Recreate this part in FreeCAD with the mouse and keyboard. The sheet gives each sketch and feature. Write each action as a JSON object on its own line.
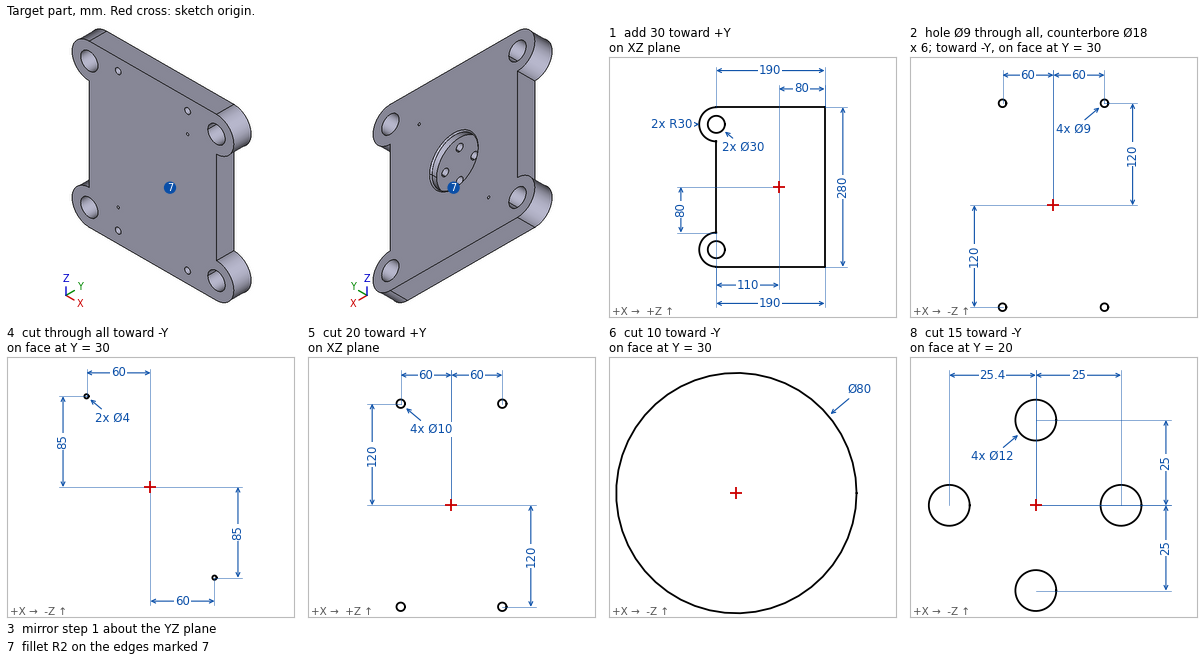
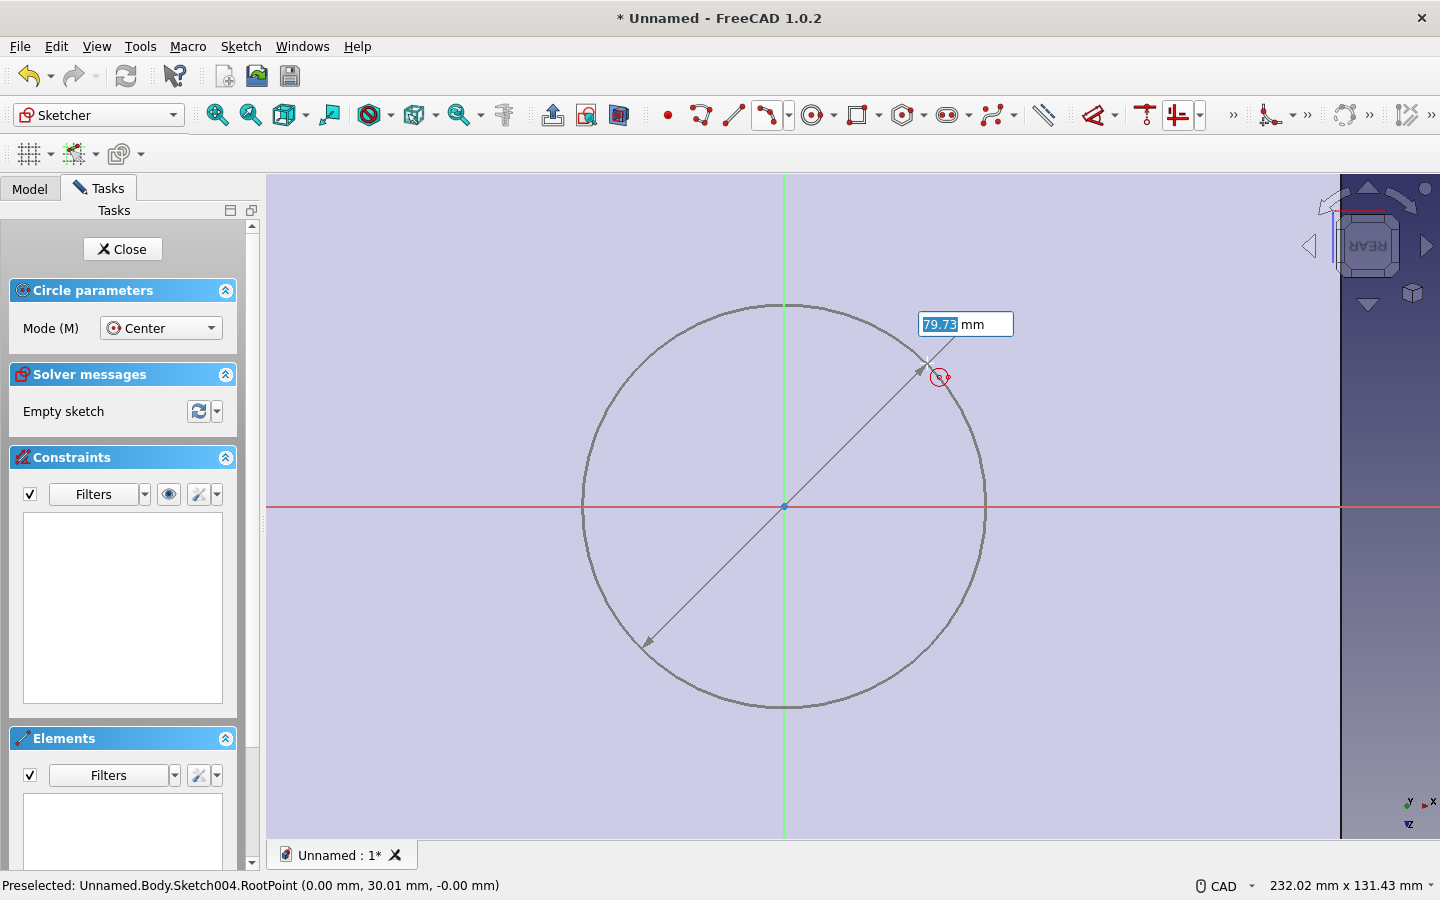
{"action": "type", "text": "80"}
{"action": "key", "text": "Return"}
{"action": "key", "text": "Escape"}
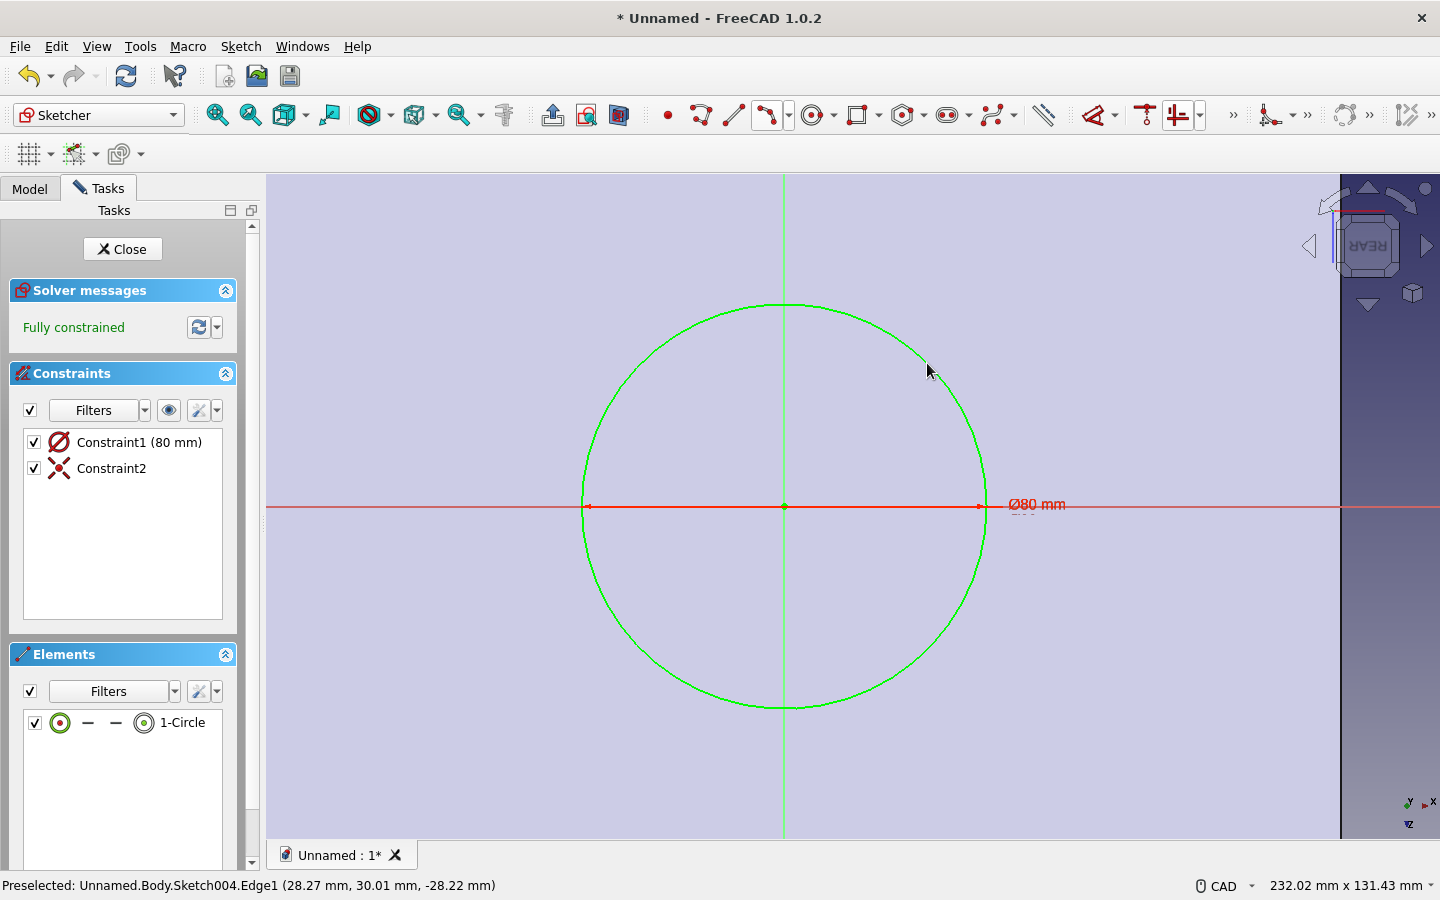
{"action": "left_click", "coordinate": [123, 249]}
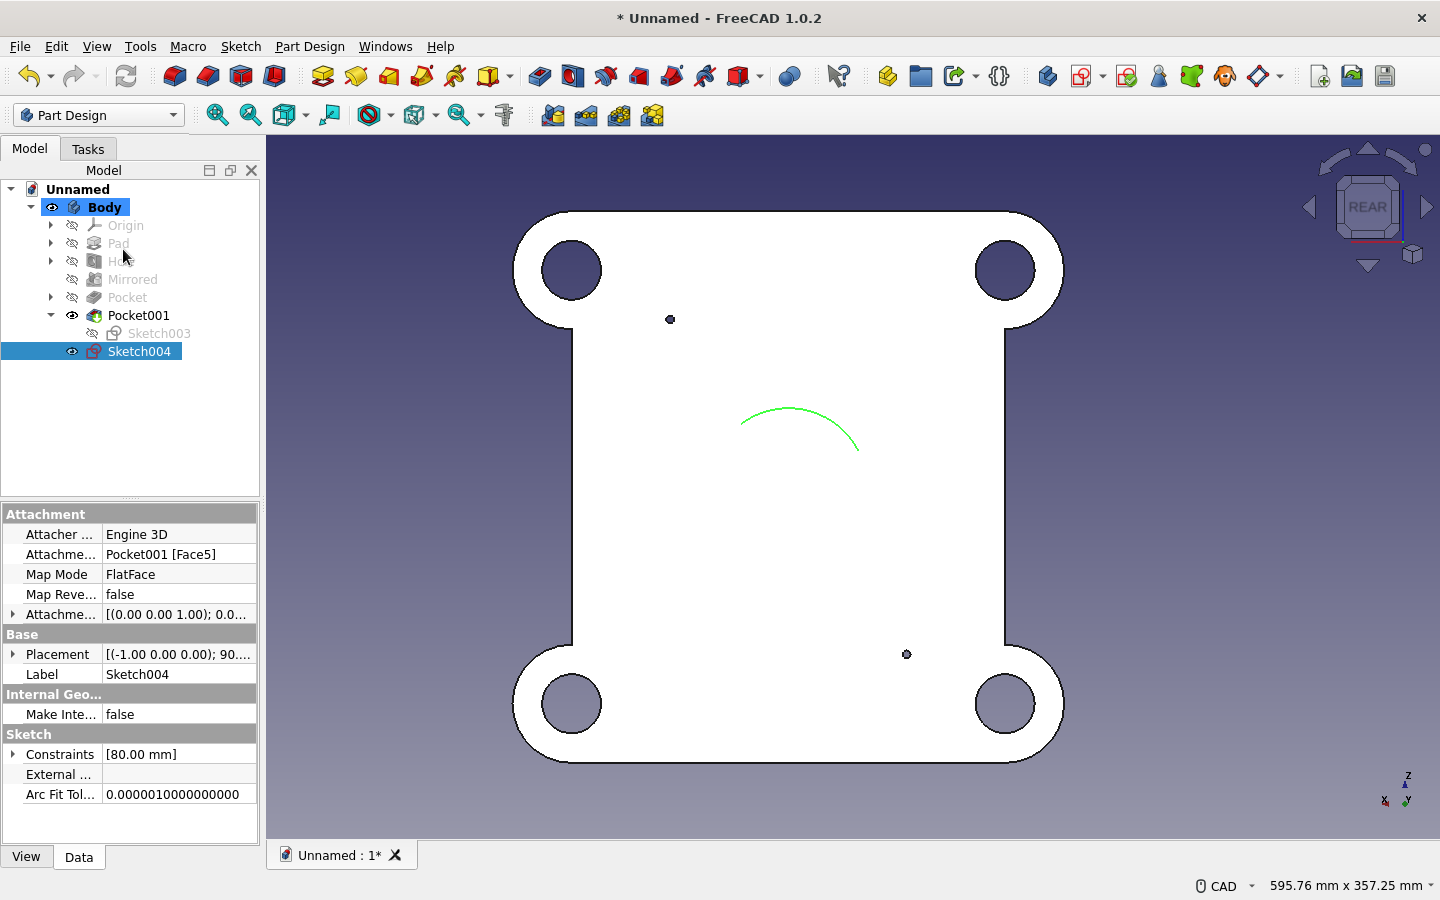
{"action": "left_click", "coordinate": [540, 76]}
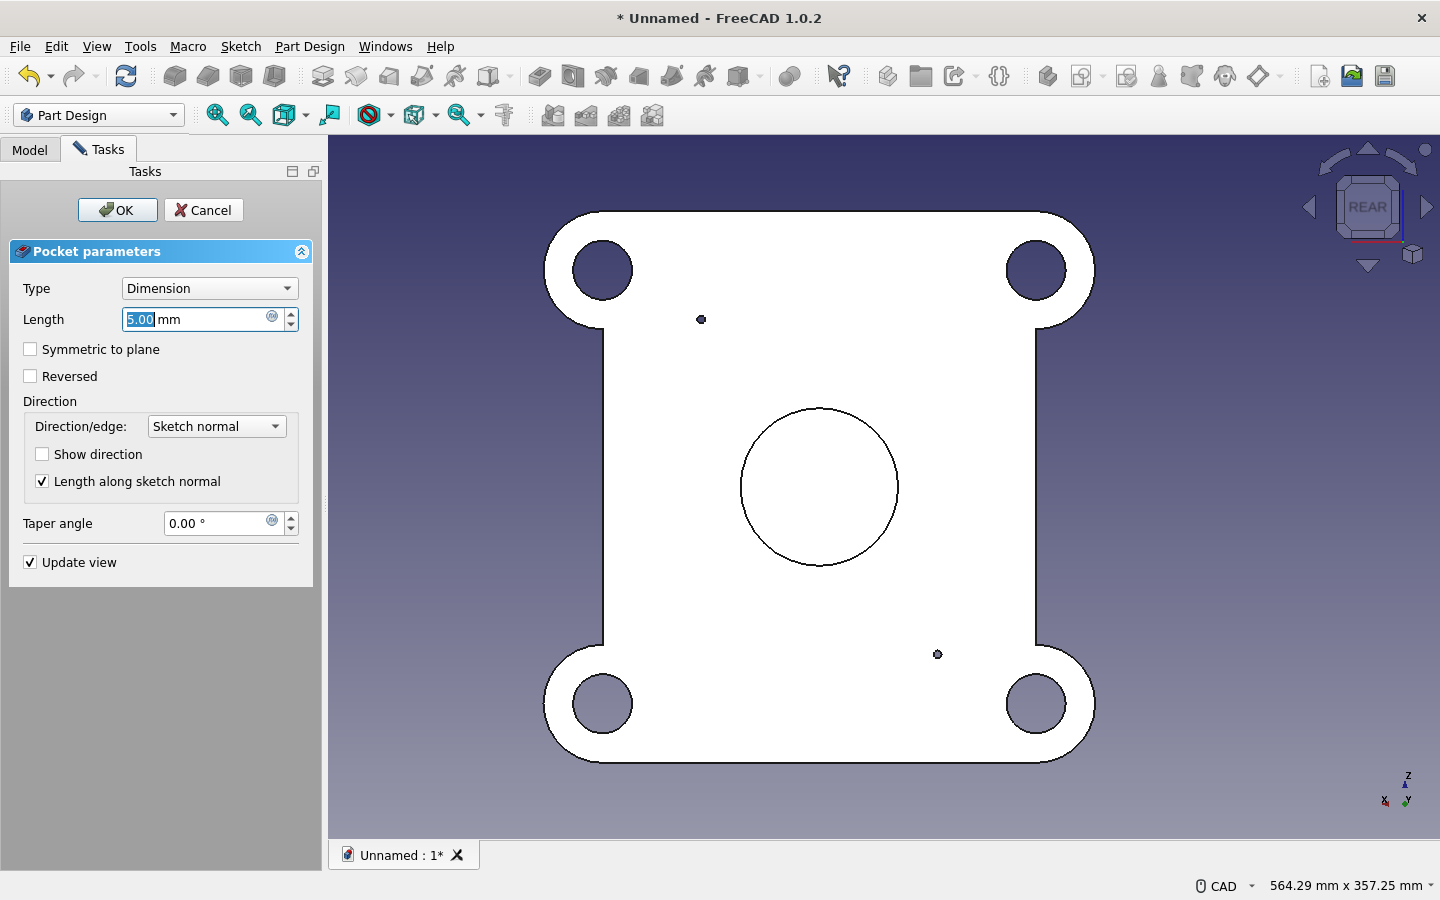
{"action": "type", "text": "10"}
{"action": "key", "text": "Tab"}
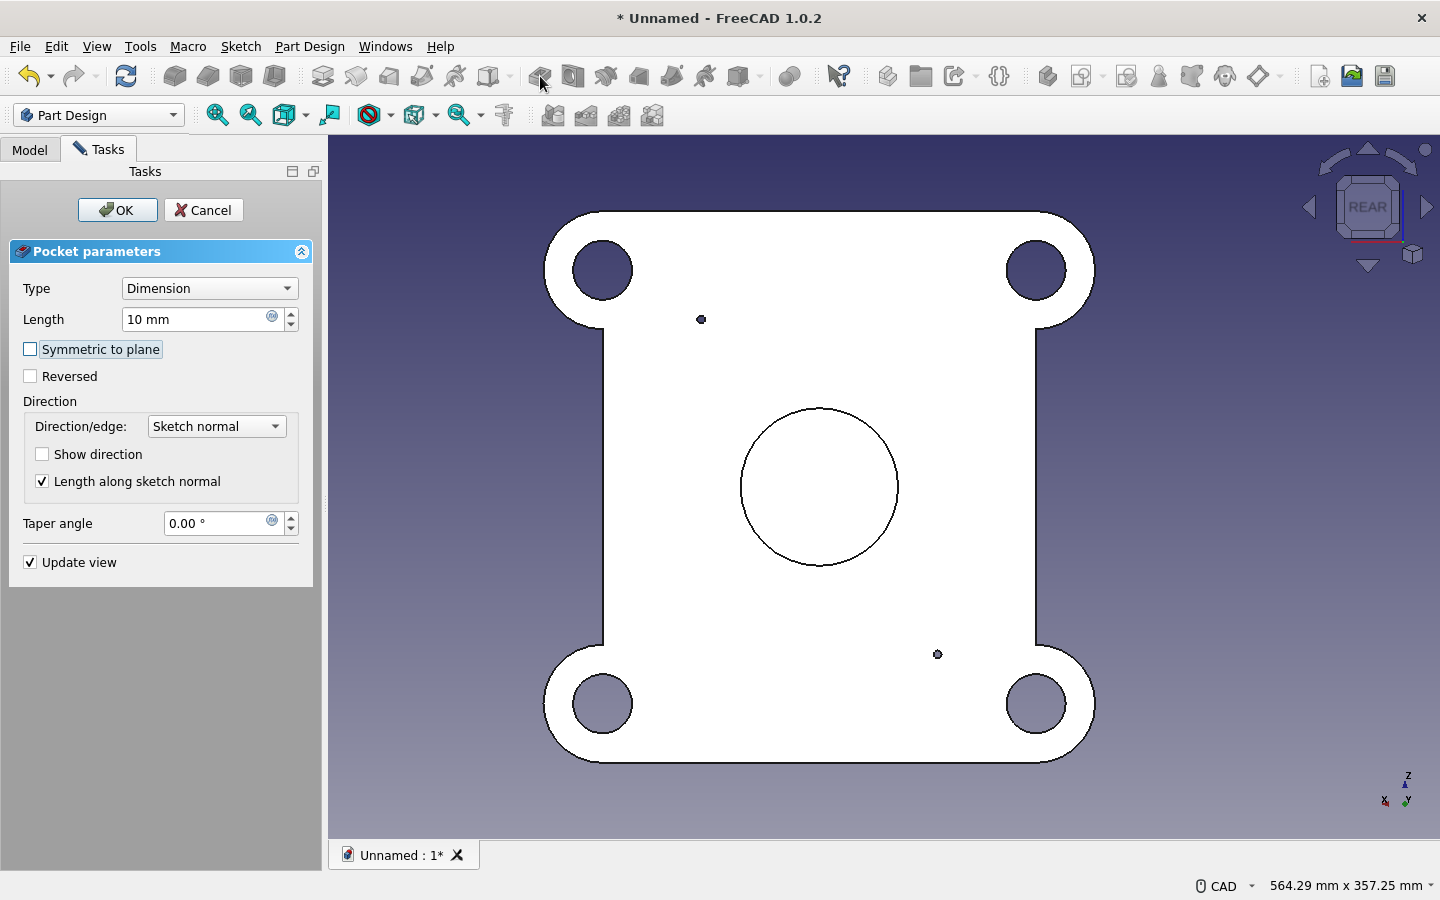
{"action": "left_click", "coordinate": [118, 210]}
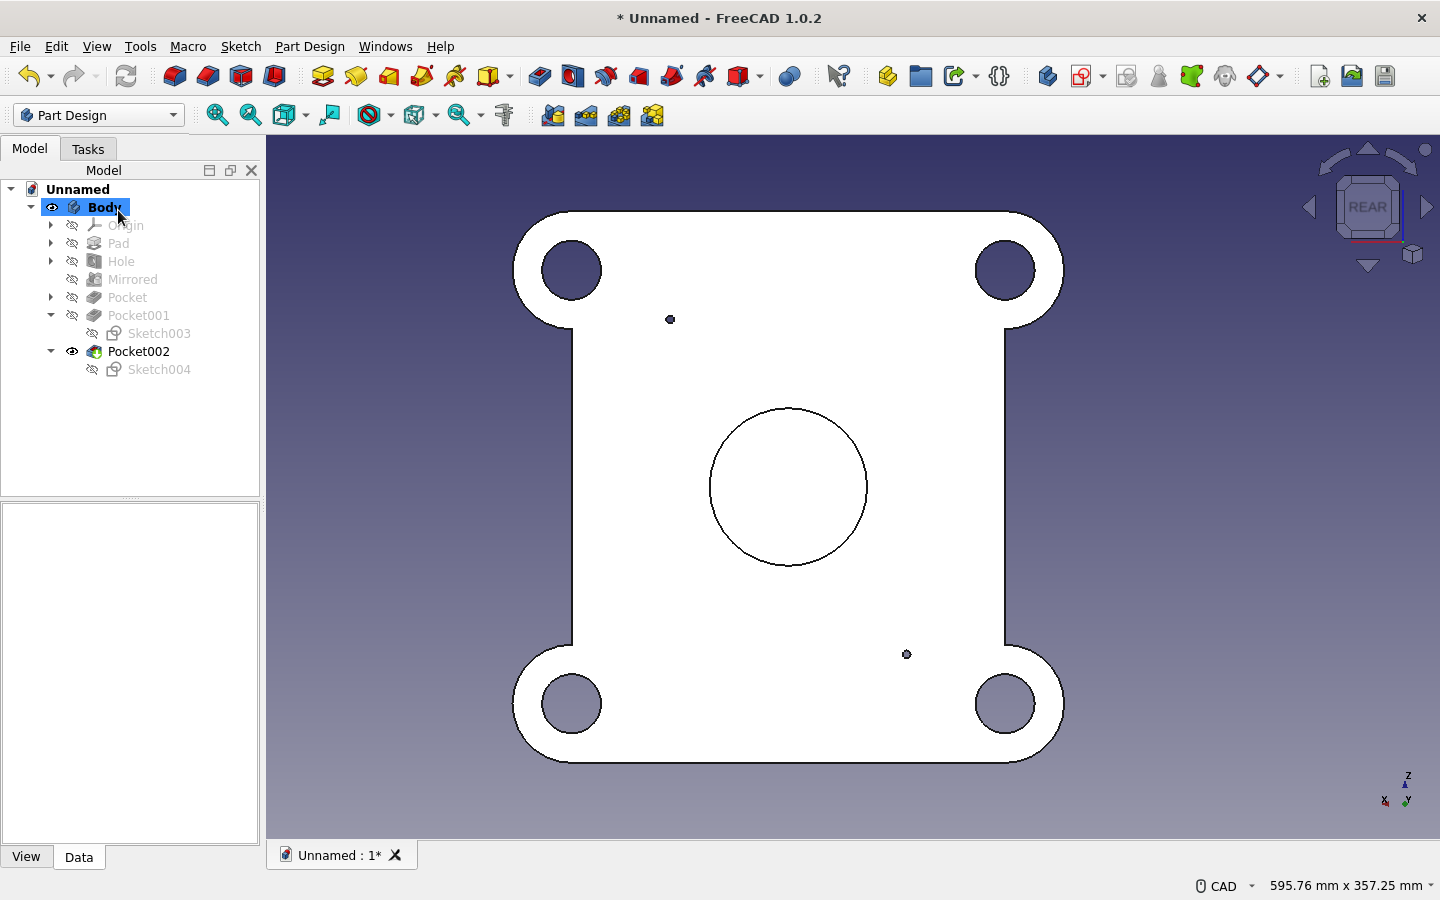
{"action": "left_click", "coordinate": [852, 440]}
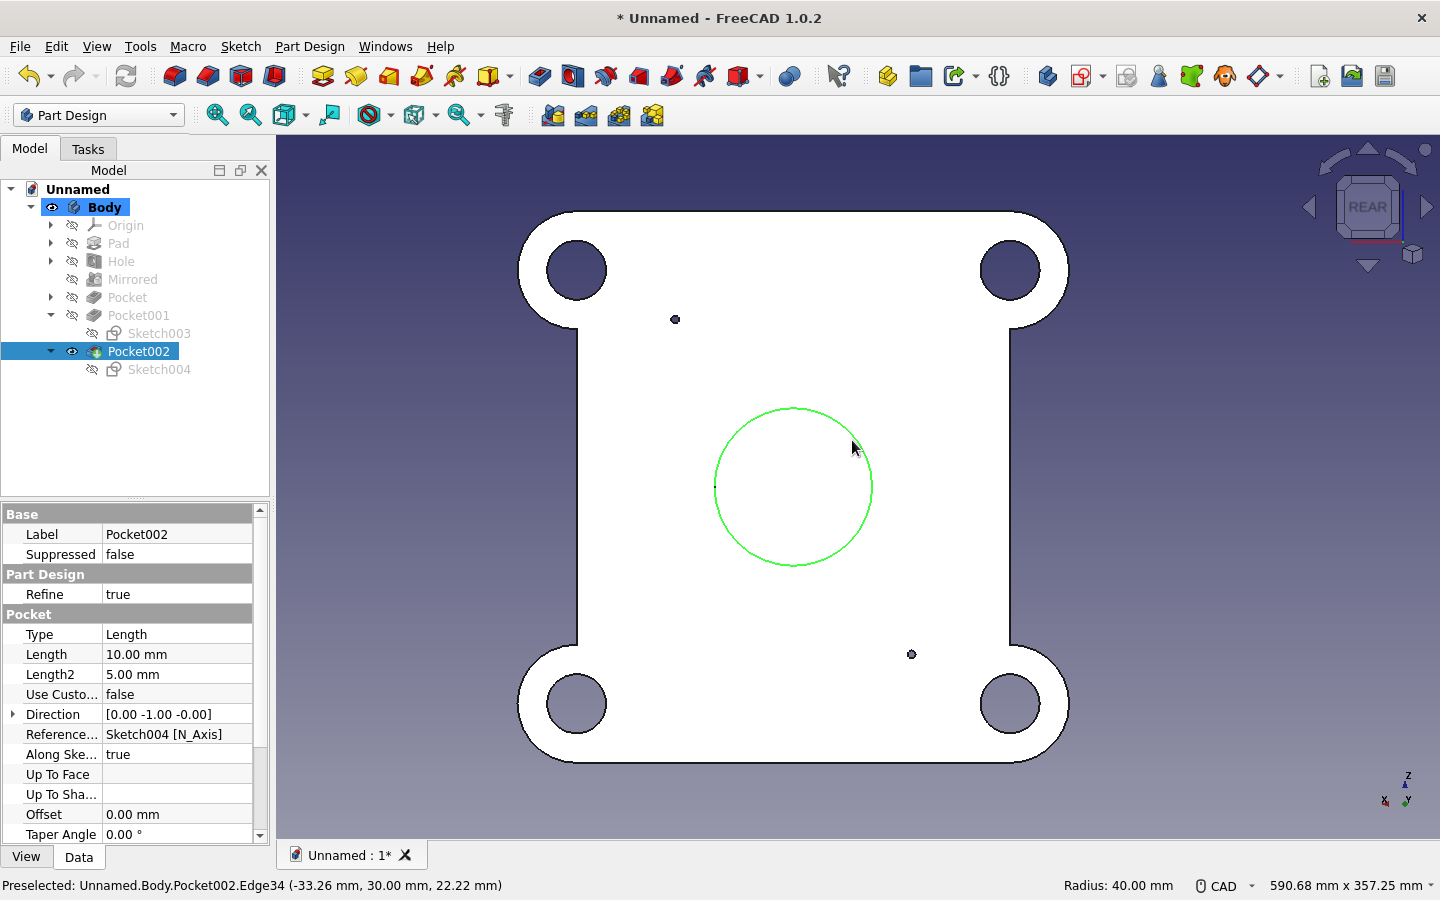
{"action": "left_click", "coordinate": [175, 76]}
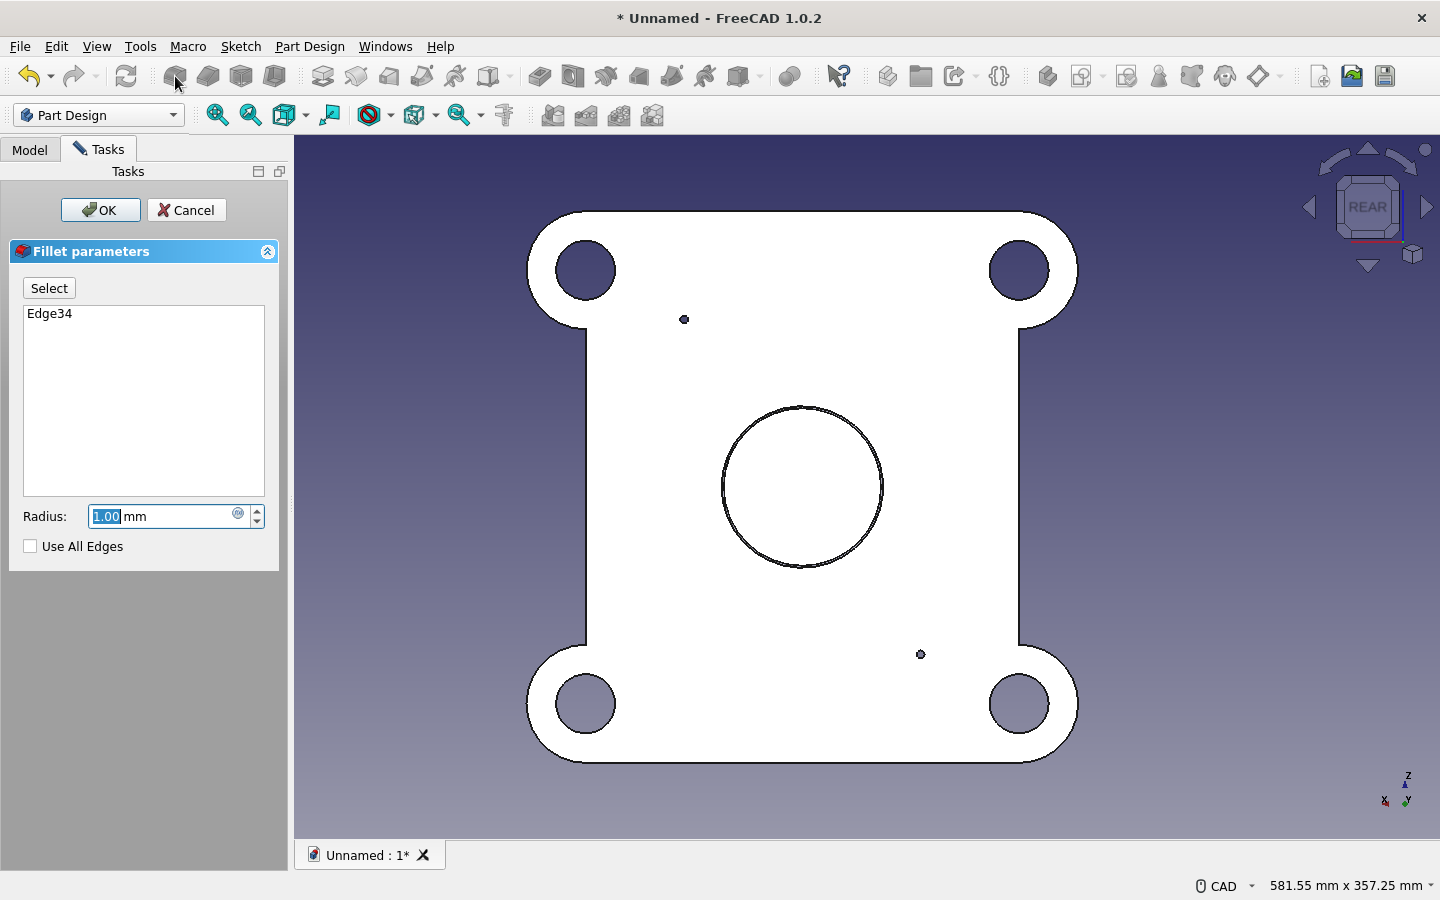
{"action": "type", "text": "2"}
{"action": "key", "text": "Tab"}